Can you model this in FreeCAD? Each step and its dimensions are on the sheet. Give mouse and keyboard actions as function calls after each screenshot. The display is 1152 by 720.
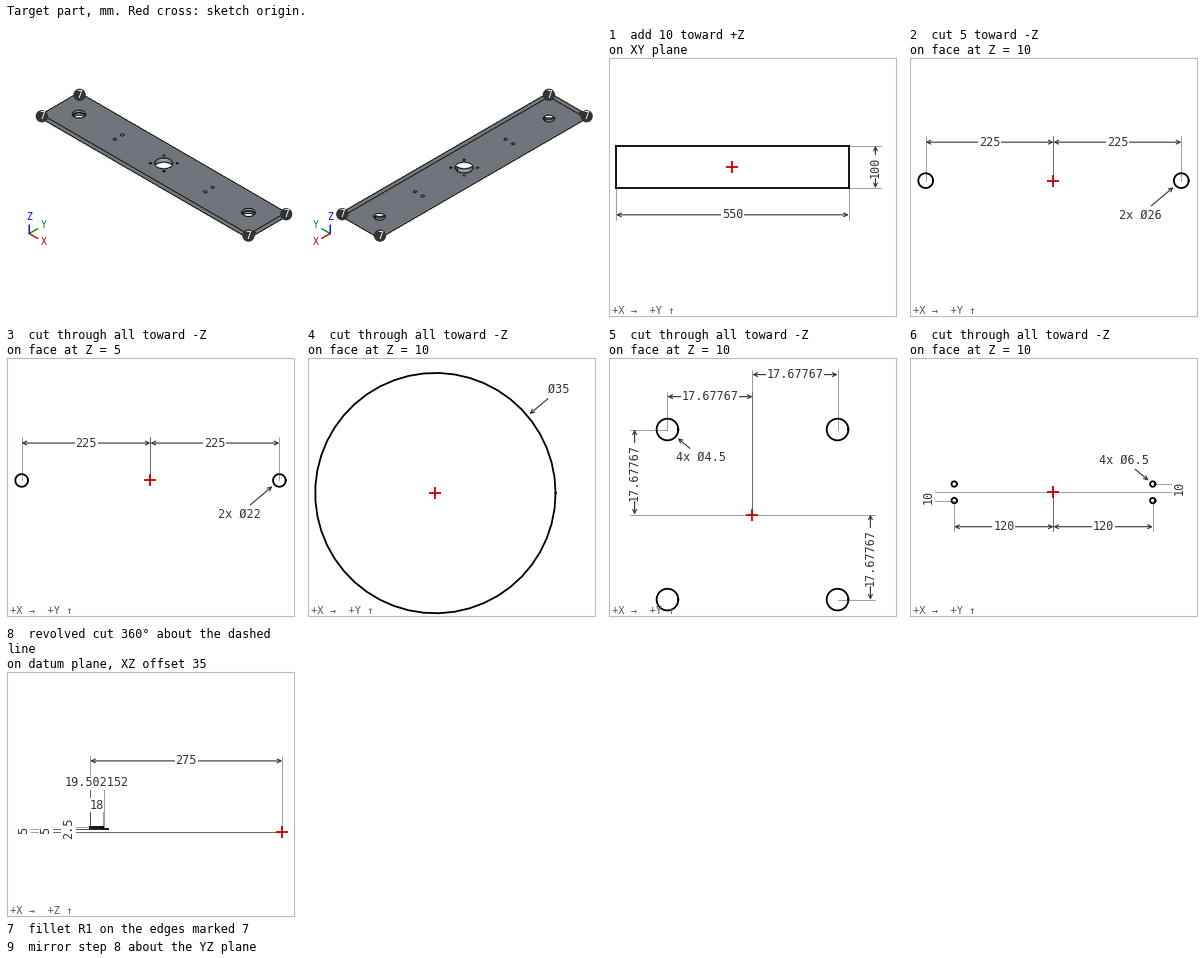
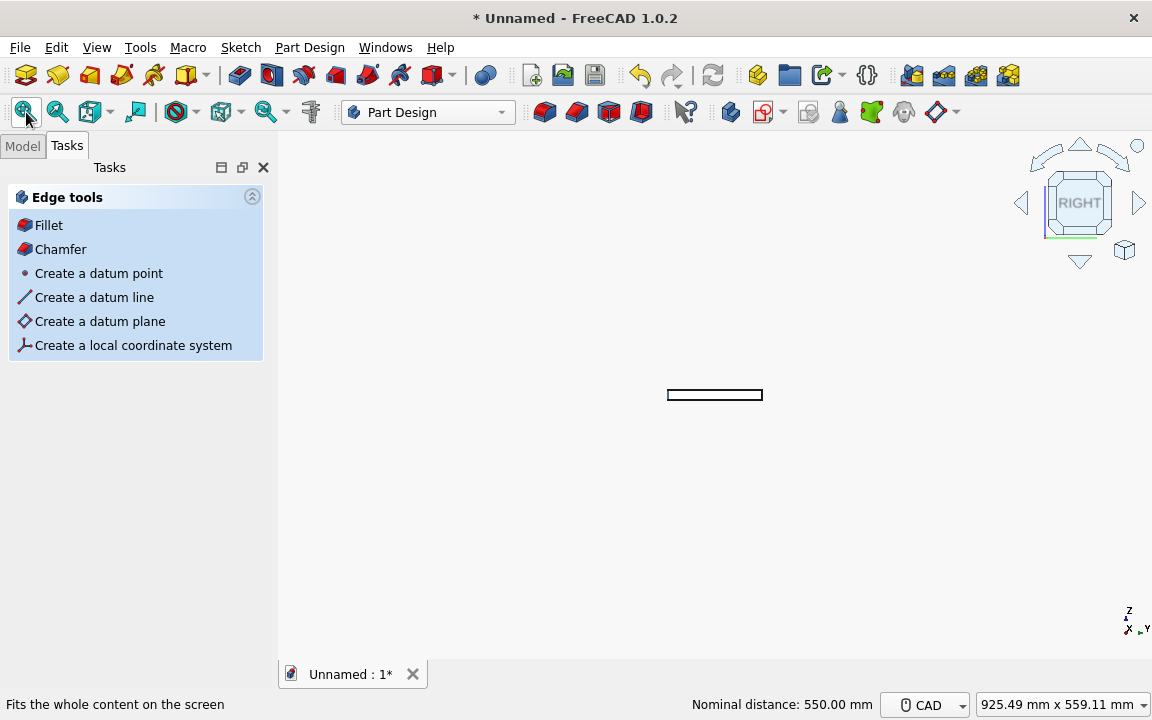
click(26, 112)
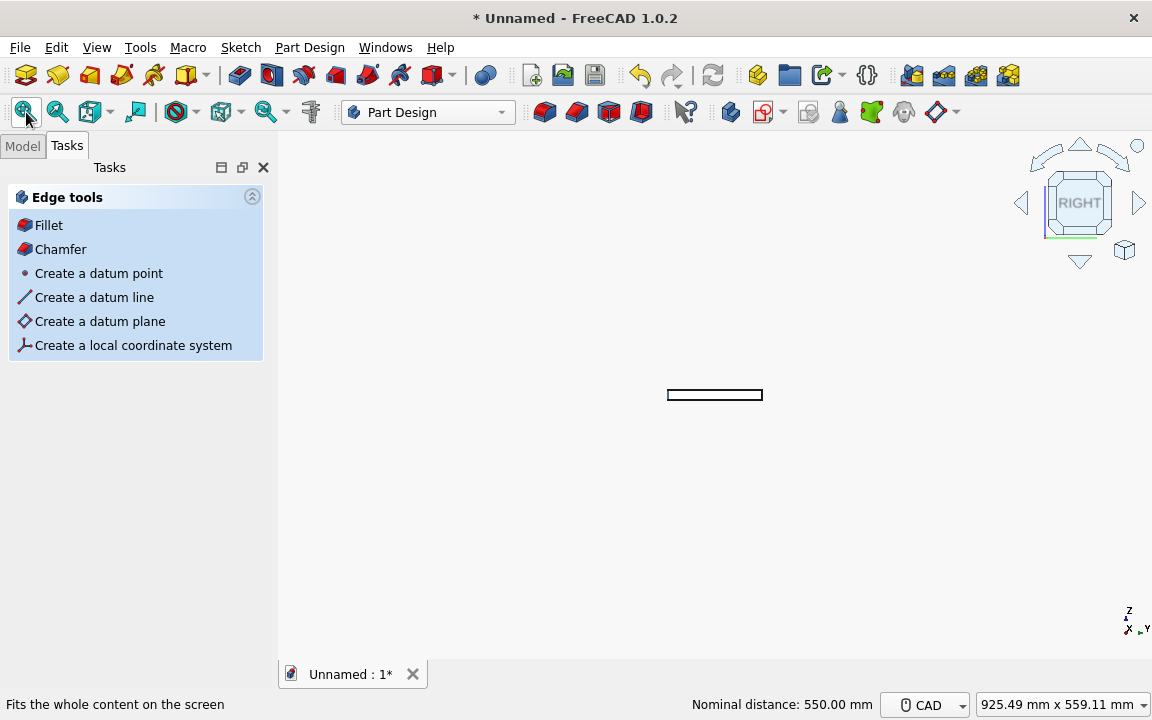
scroll(762, 394, up, 8)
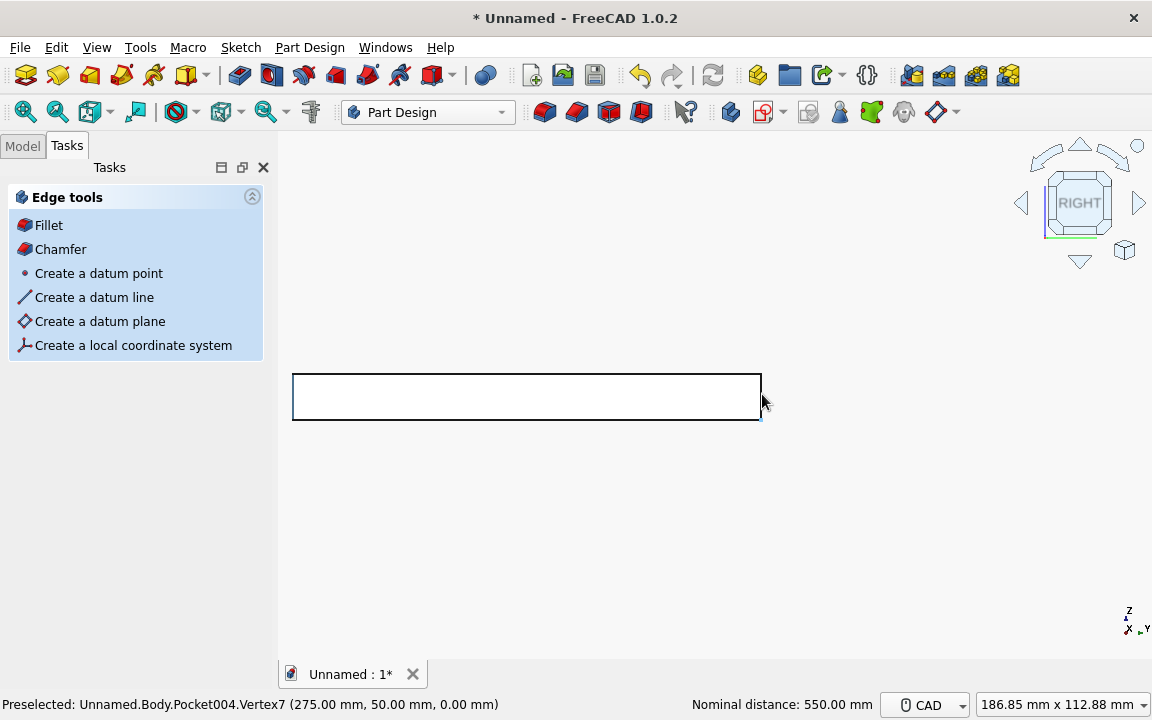
click(761, 396, ctrl)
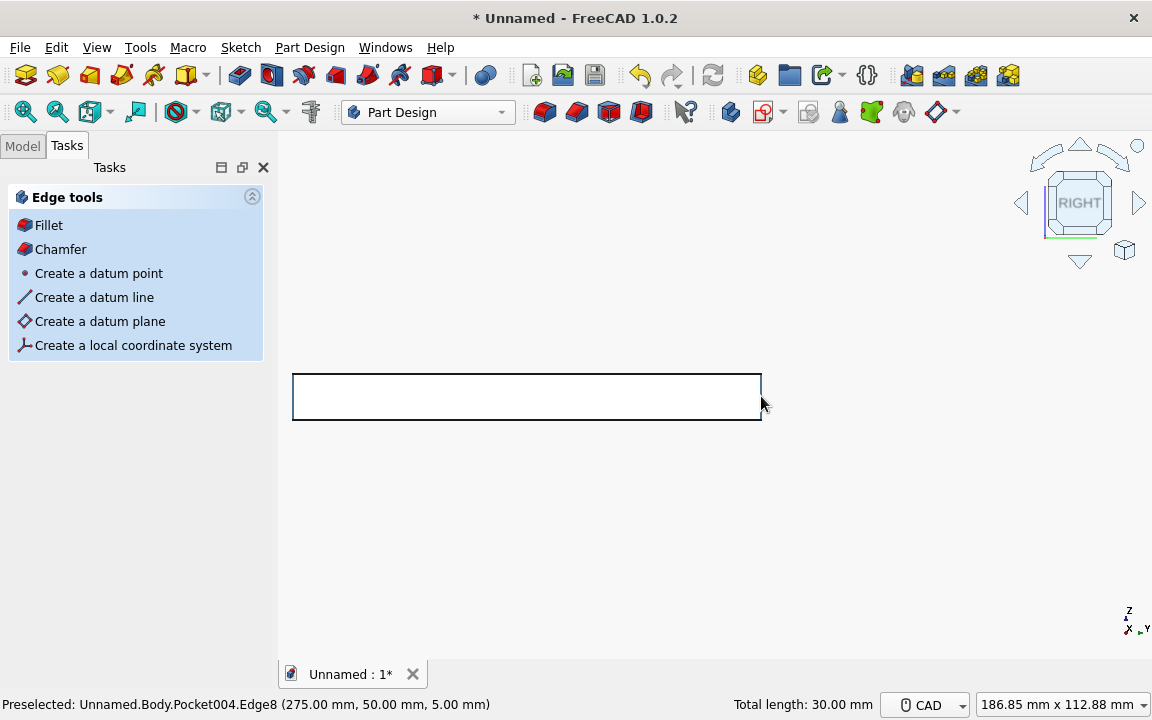
click(26, 112)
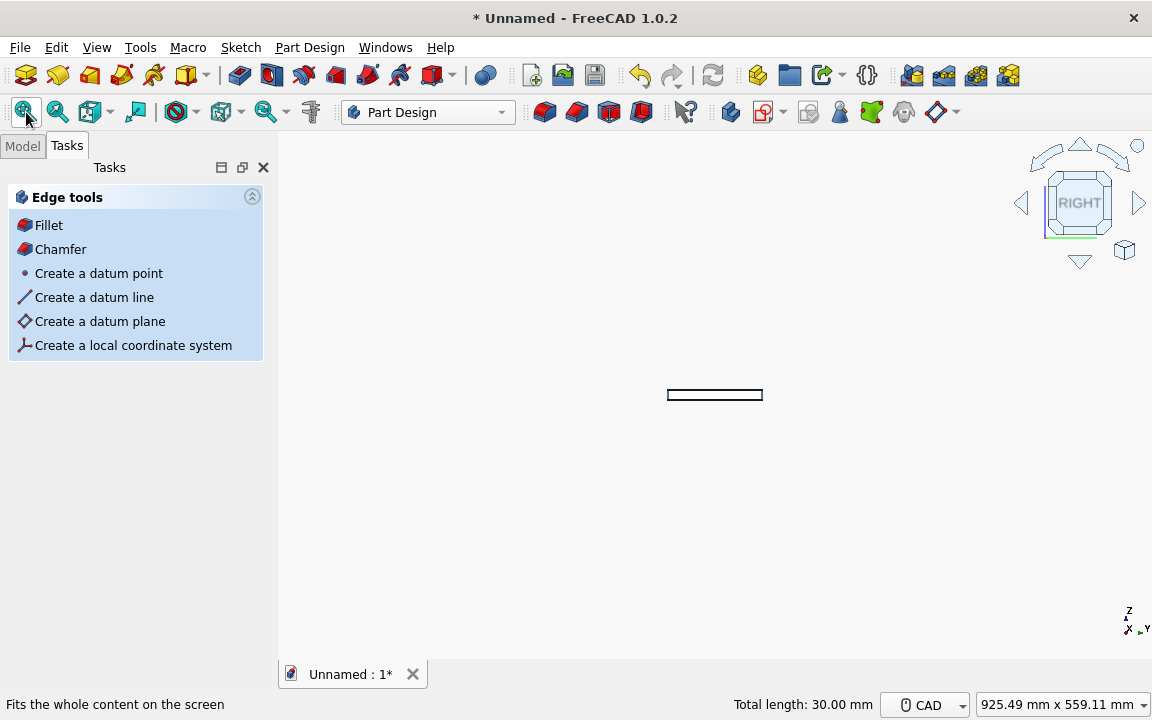
key(5)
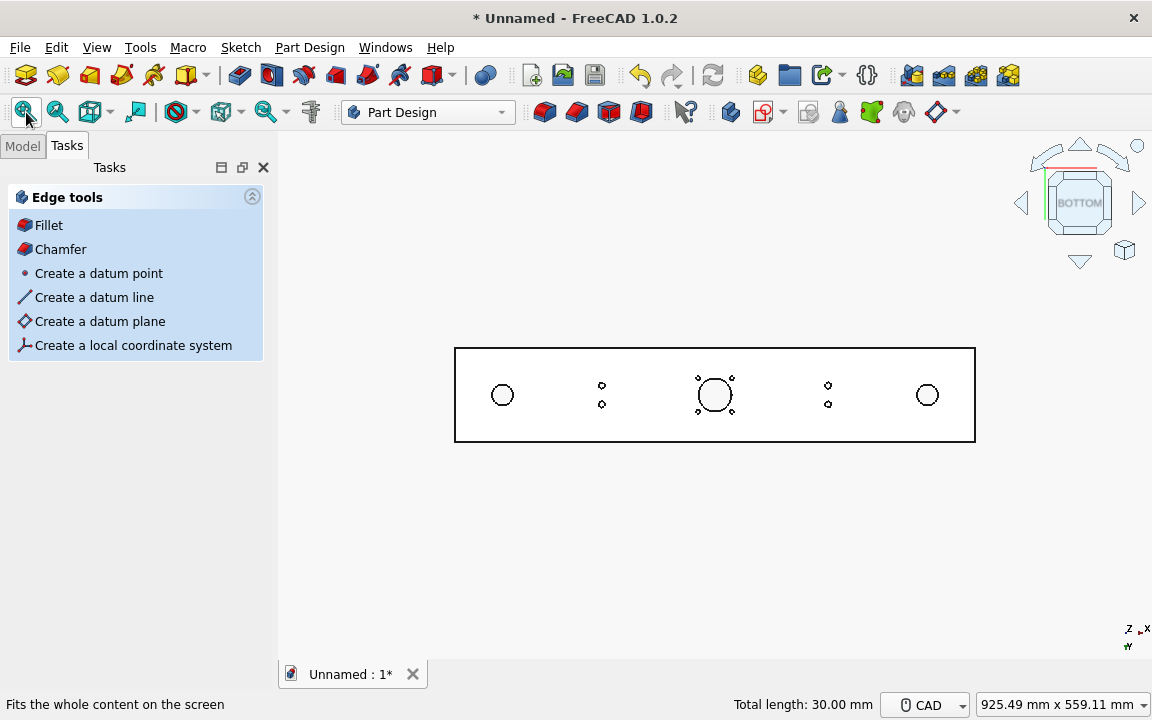
scroll(455, 441, up, 8)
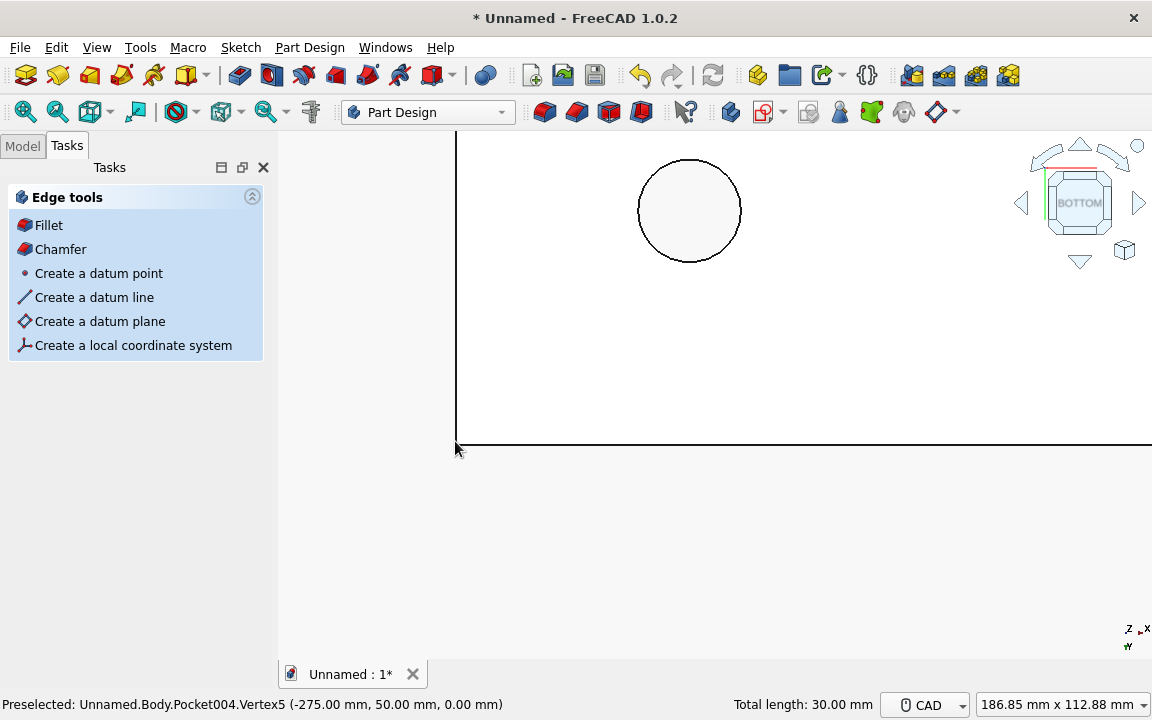
click(26, 112)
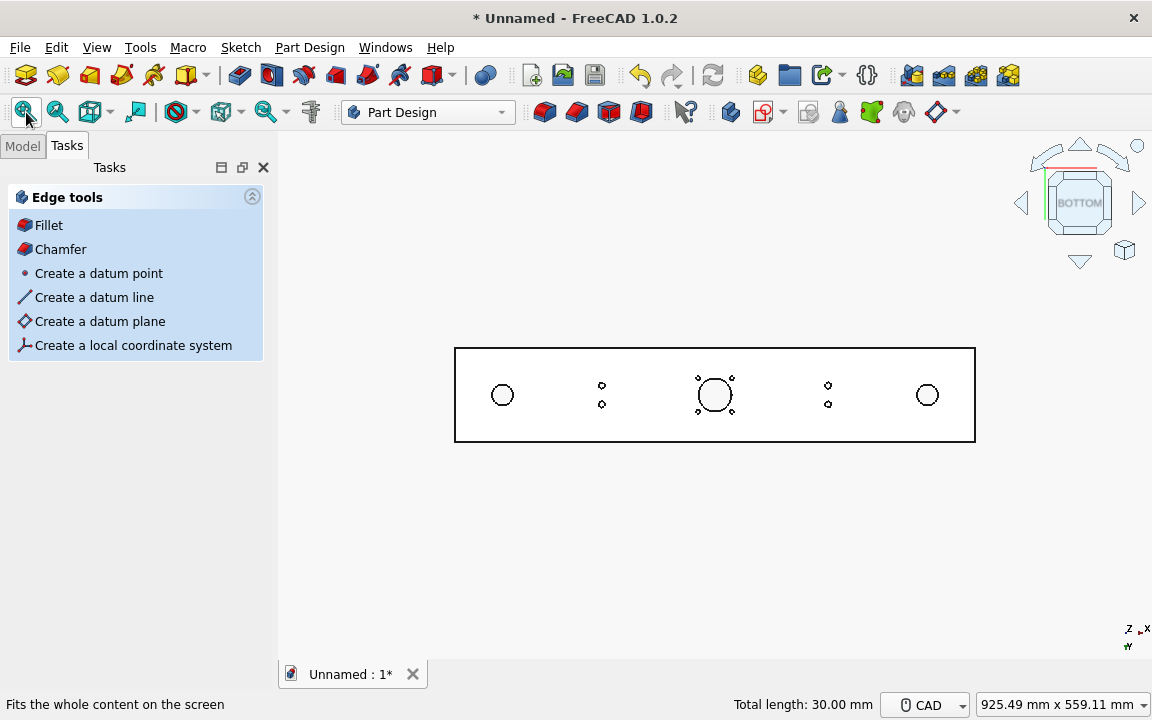
key(4)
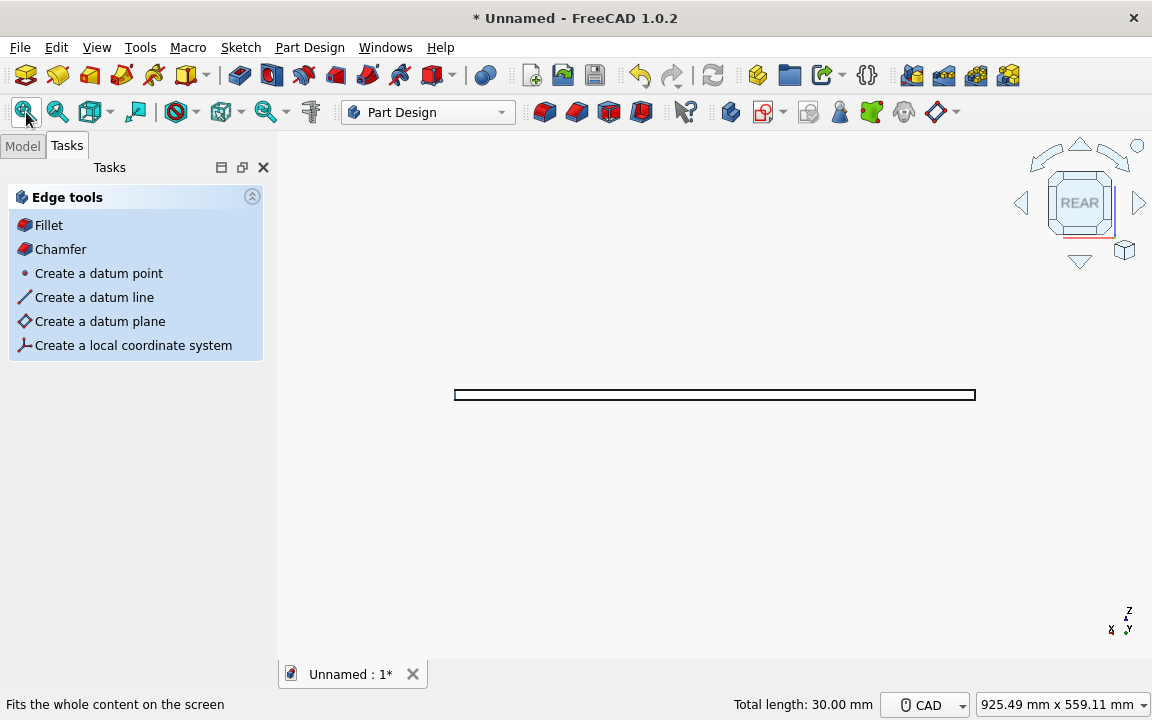
scroll(975, 394, up, 8)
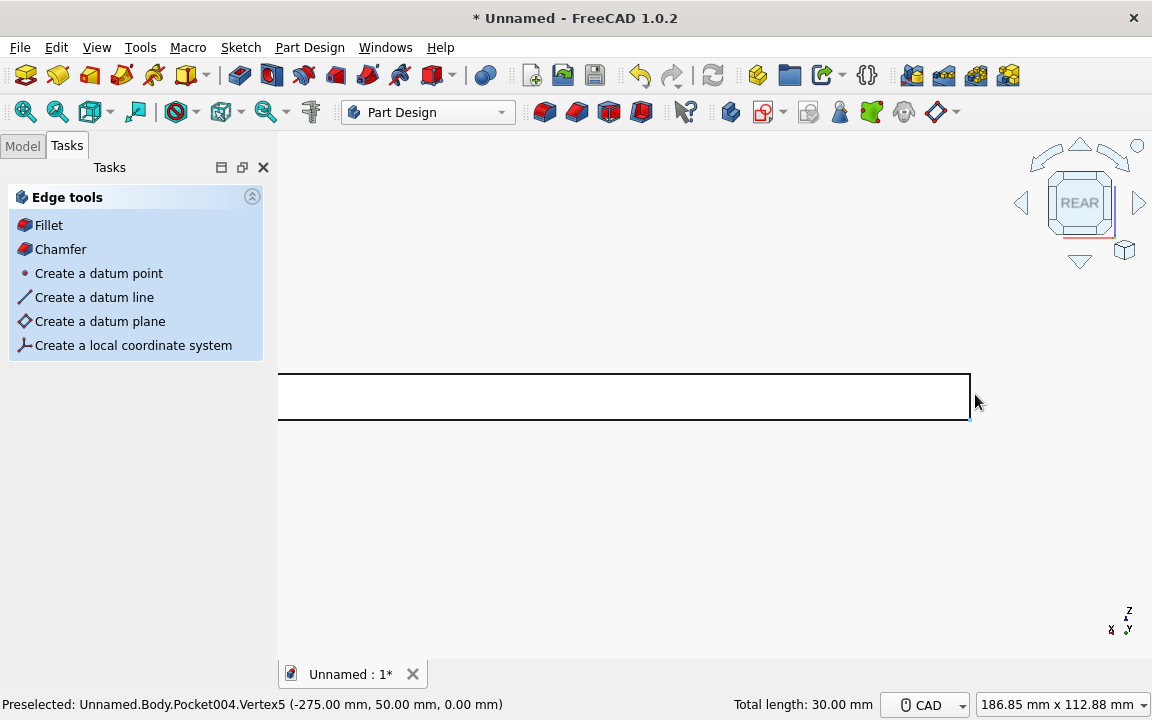
click(970, 396, ctrl)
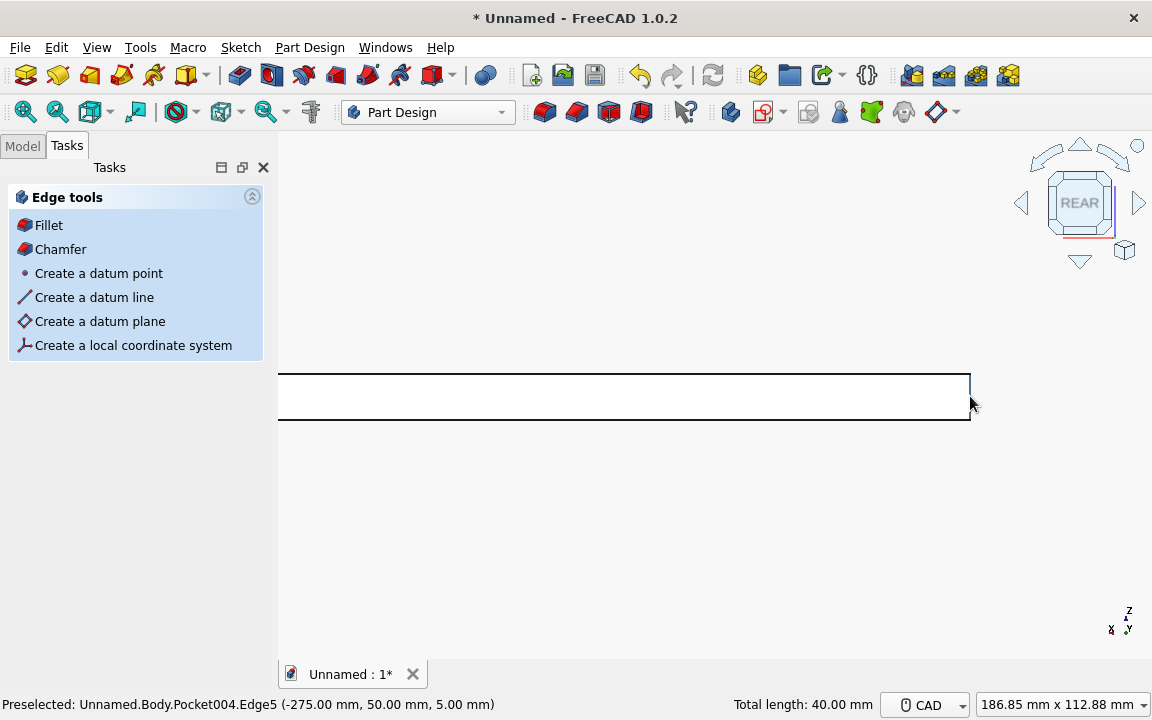
click(546, 112)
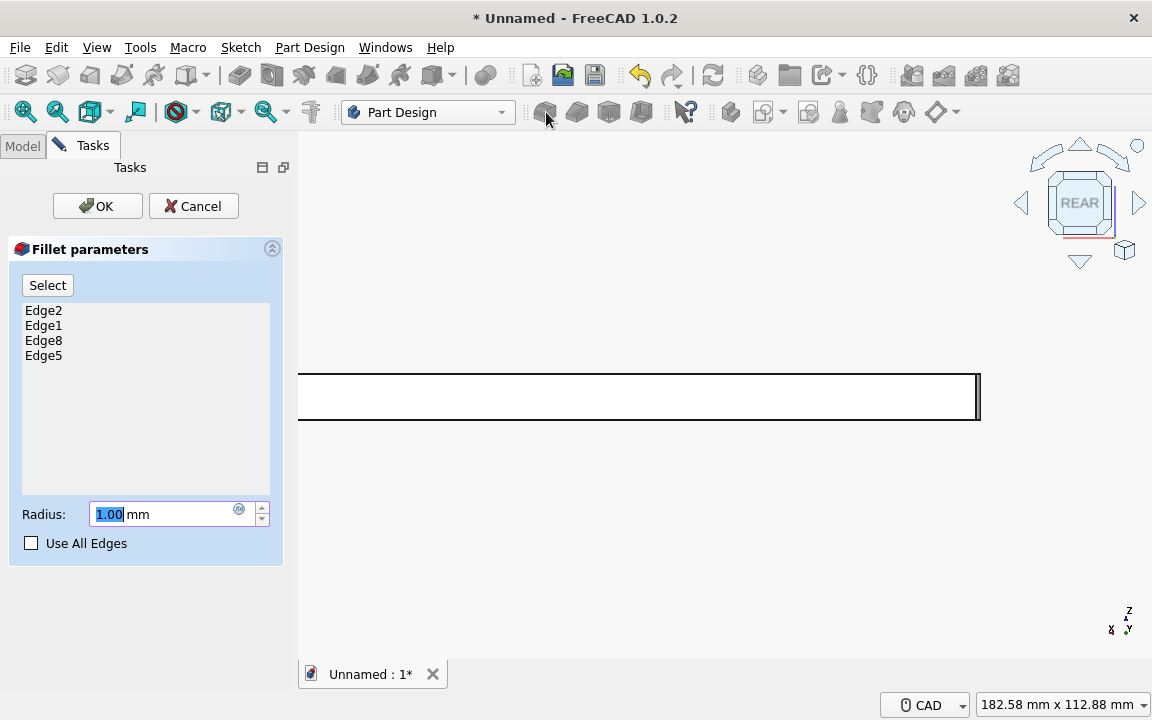
text(1)
key(Tab)